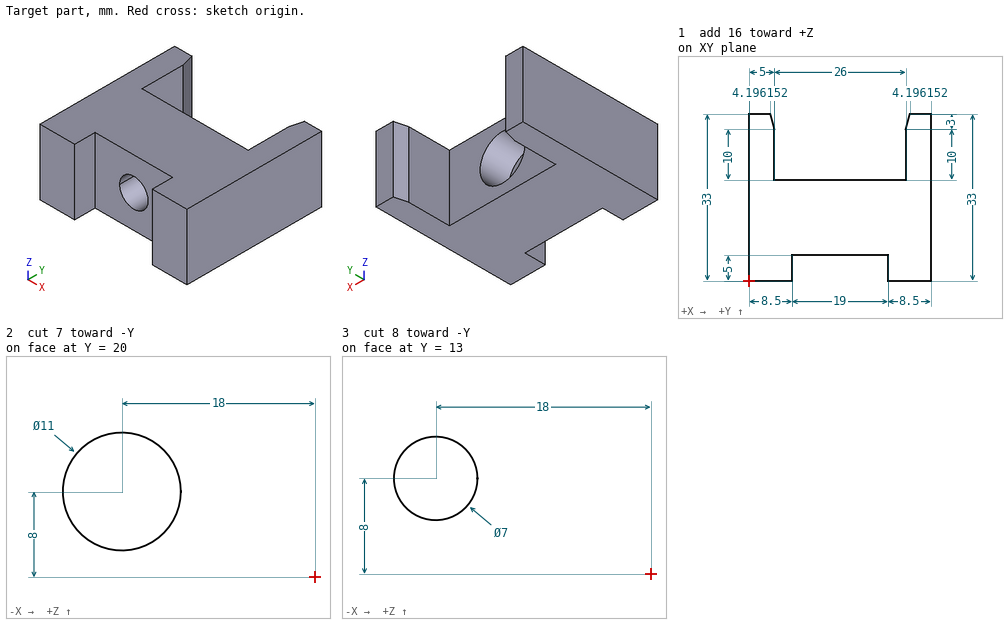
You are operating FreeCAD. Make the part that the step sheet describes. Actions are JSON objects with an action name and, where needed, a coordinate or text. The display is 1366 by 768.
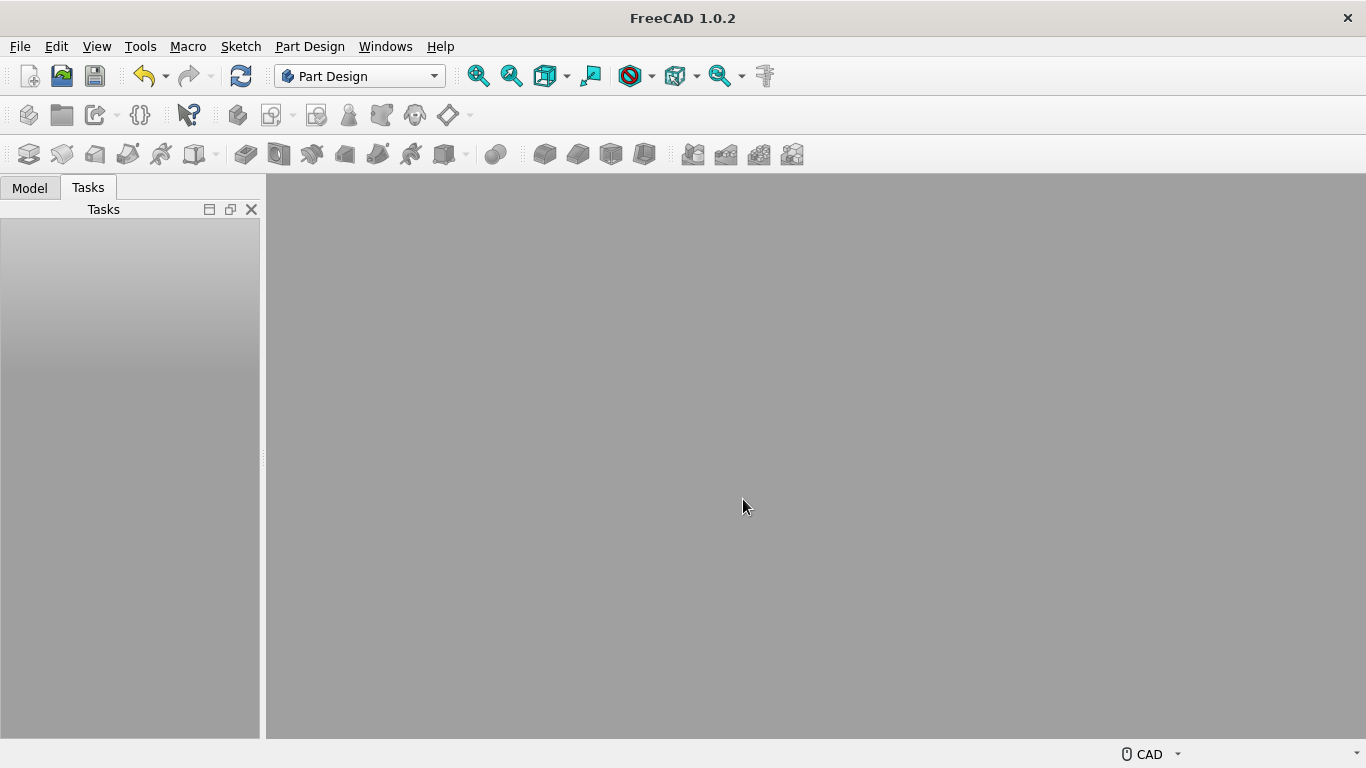
{"action": "left_click", "coordinate": [29, 76]}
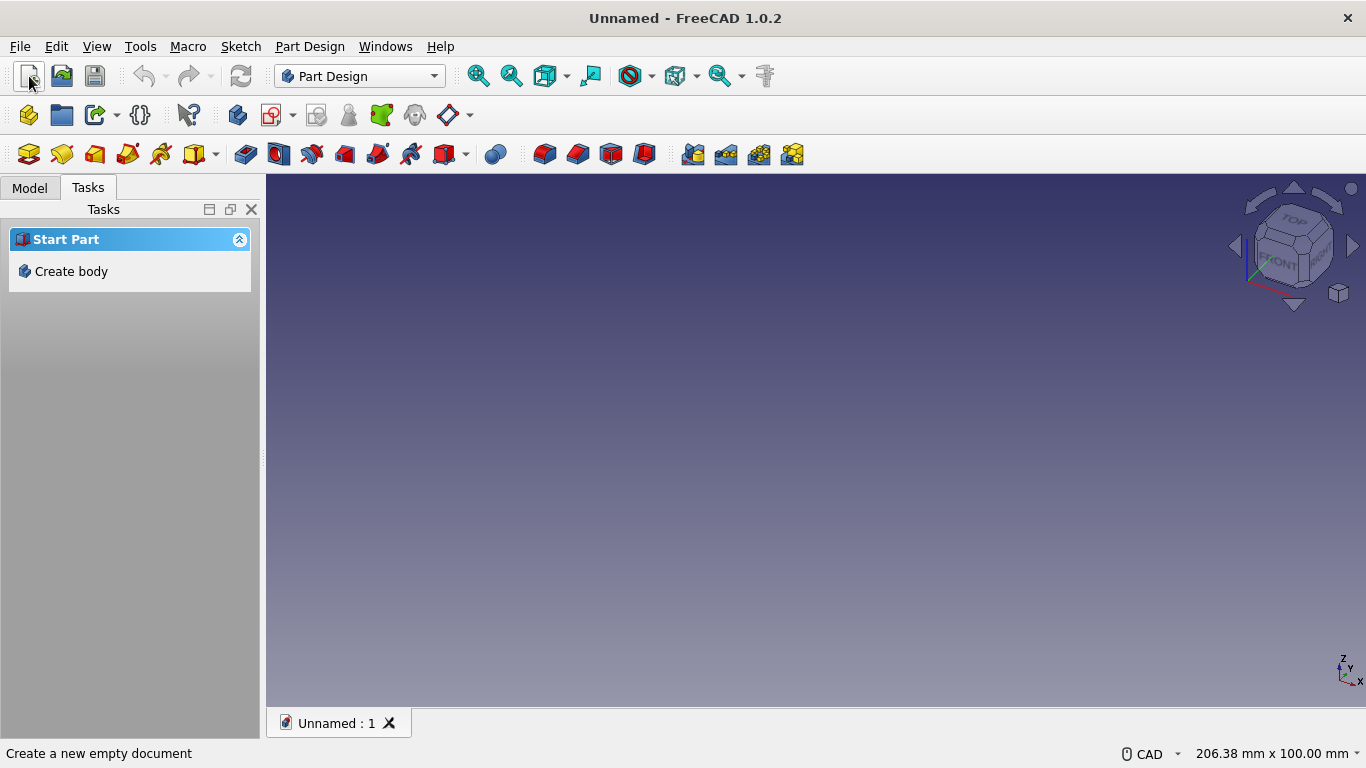
{"action": "left_click", "coordinate": [270, 116]}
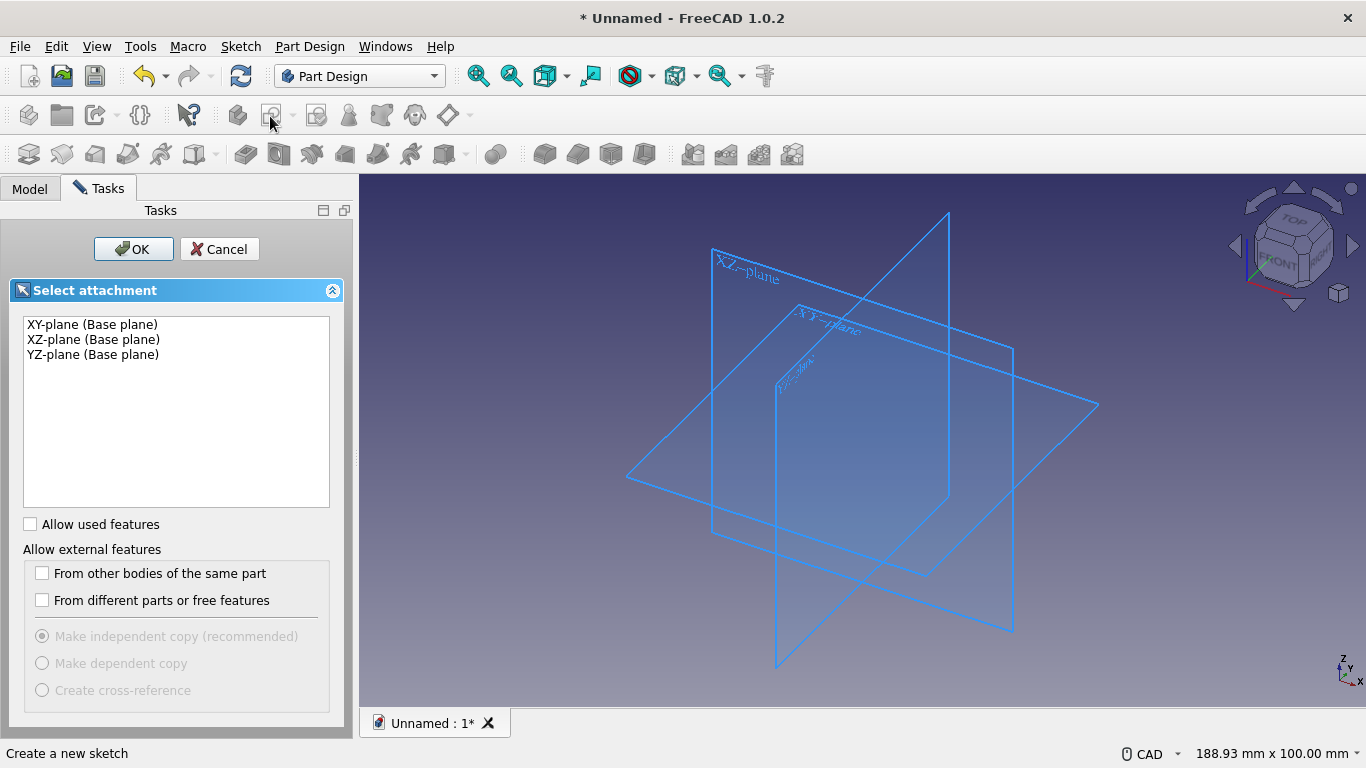
{"action": "left_click", "coordinate": [84, 324]}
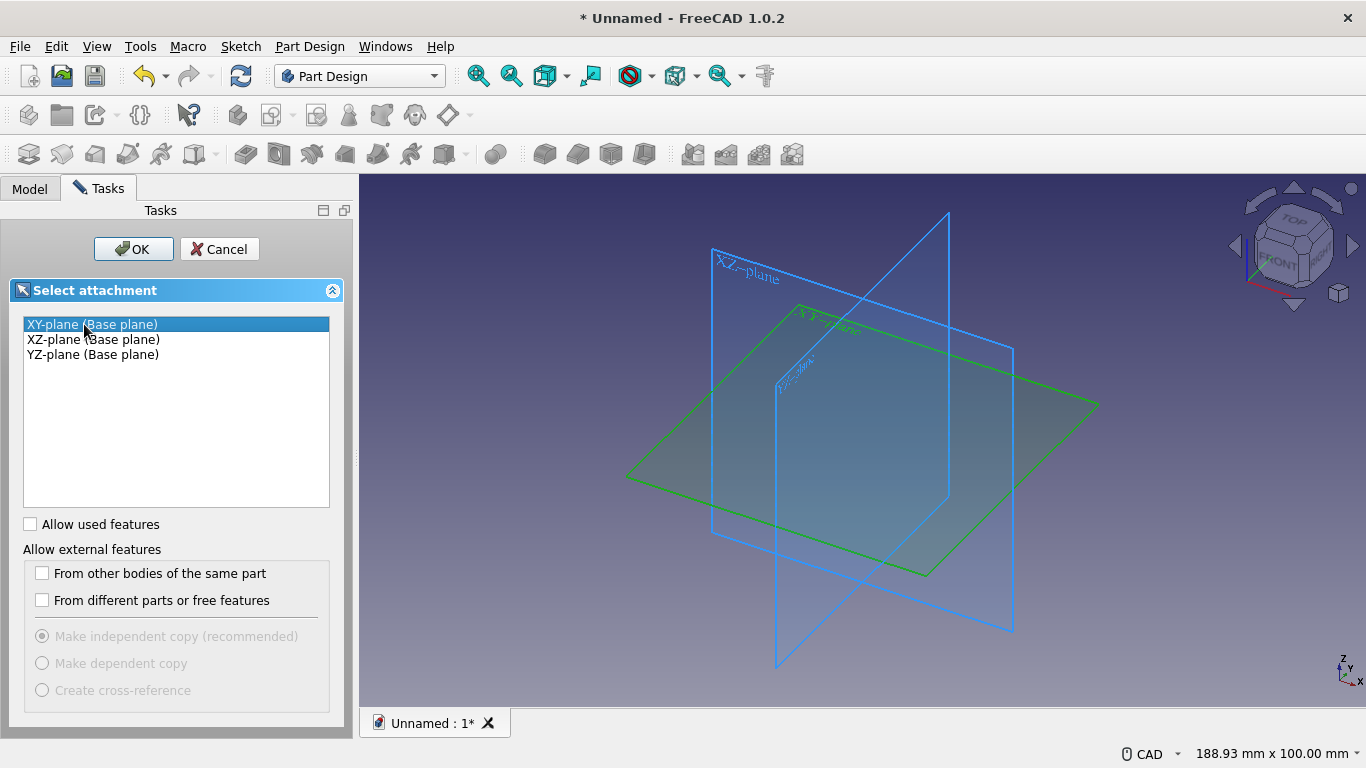
{"action": "left_click", "coordinate": [134, 249]}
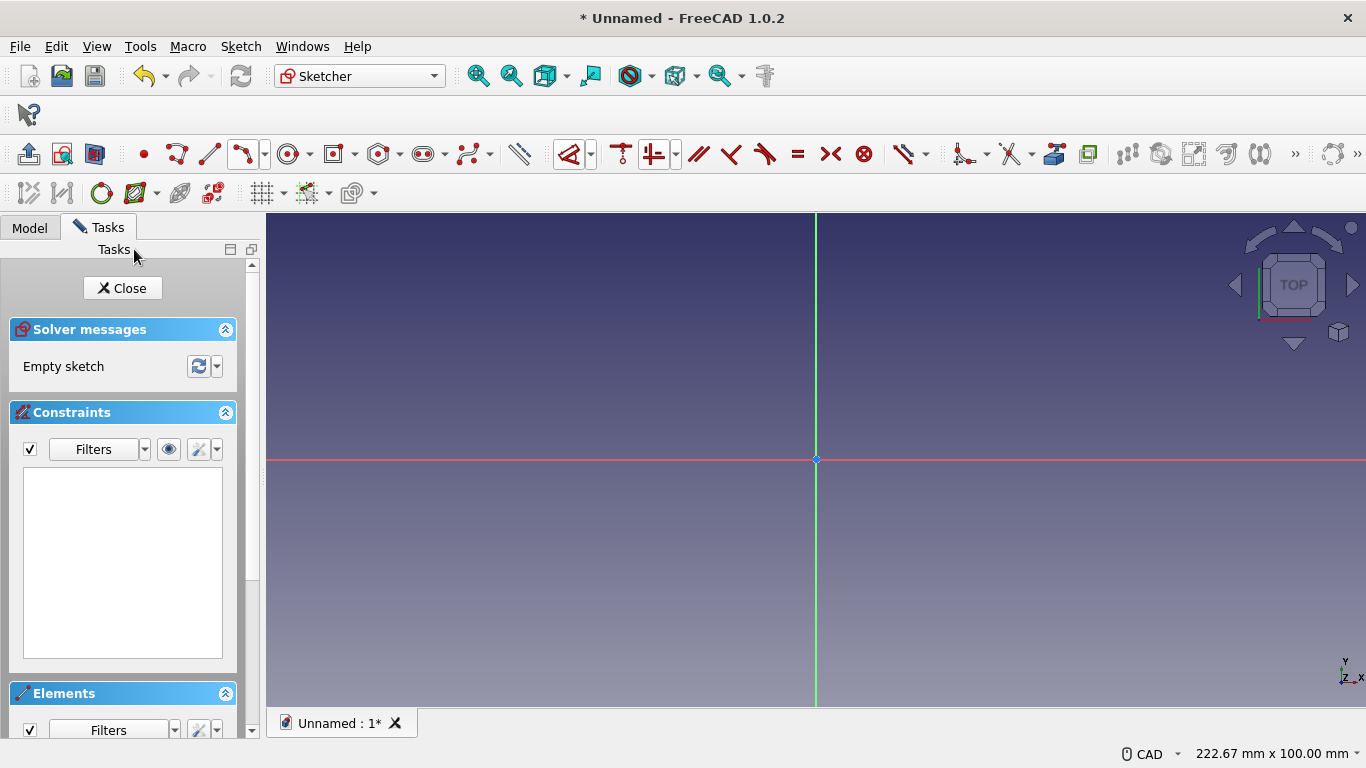
{"action": "scroll", "coordinate": [1096, 279], "scroll_direction": "up", "scroll_amount": 3}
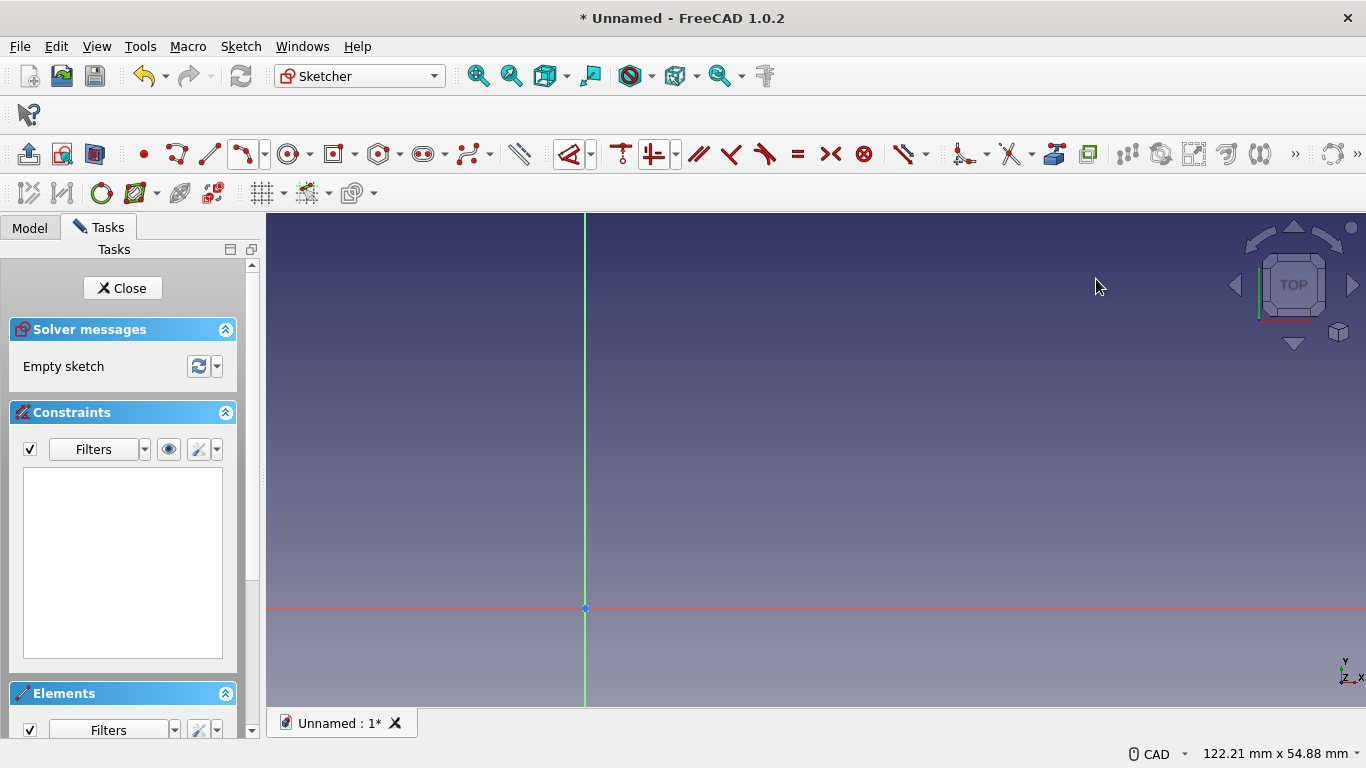
{"action": "left_click", "coordinate": [177, 154]}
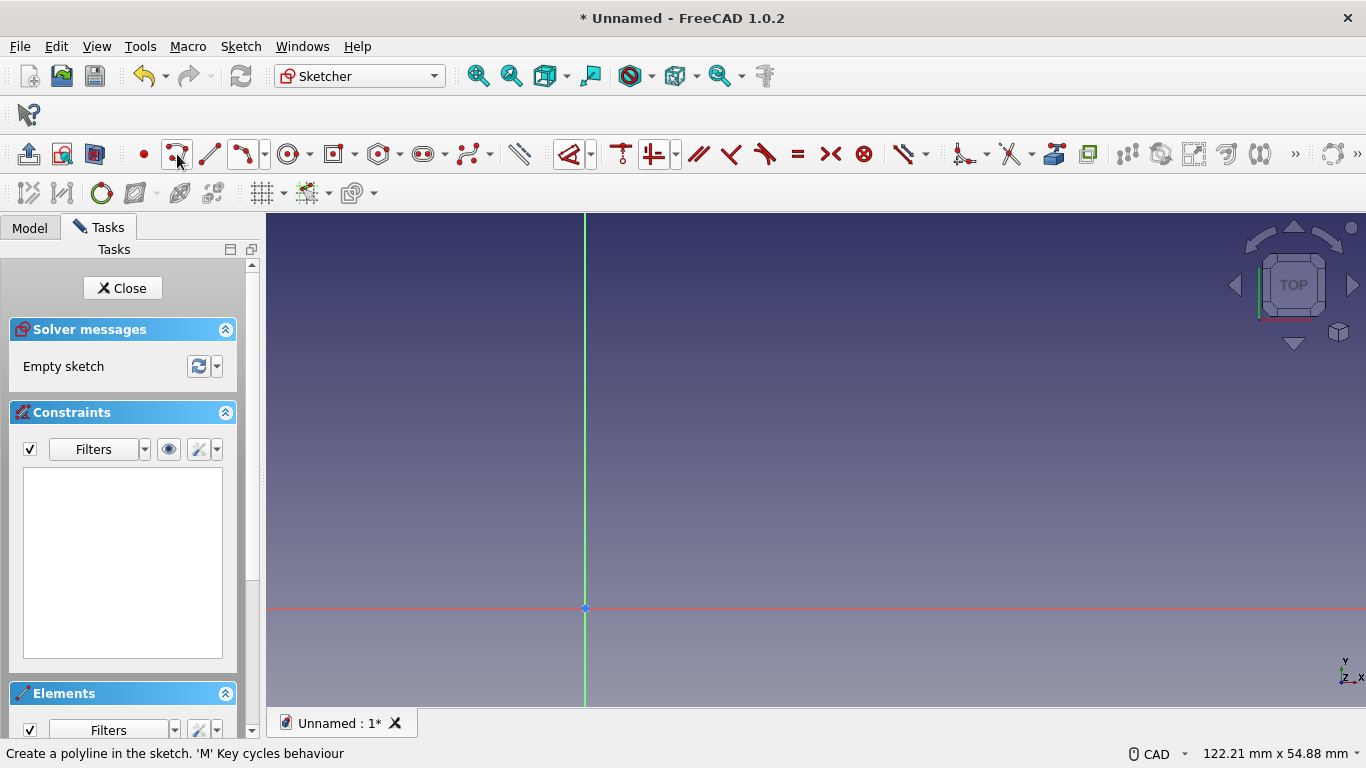
{"action": "left_click", "coordinate": [585, 609]}
{"action": "left_click", "coordinate": [662, 600]}
{"action": "left_click", "coordinate": [662, 564]}
{"action": "left_click", "coordinate": [833, 564]}
{"action": "left_click", "coordinate": [833, 609]}
{"action": "left_click", "coordinate": [909, 600]}
{"action": "left_click", "coordinate": [909, 312]}
{"action": "left_click", "coordinate": [871, 312]}
{"action": "left_click", "coordinate": [864, 339]}
{"action": "left_click", "coordinate": [864, 429]}
{"action": "left_click", "coordinate": [630, 429]}
{"action": "left_click", "coordinate": [630, 339]}
{"action": "left_click", "coordinate": [623, 312]}
{"action": "left_click", "coordinate": [594, 312]}
{"action": "left_click", "coordinate": [585, 609]}
{"action": "key", "text": "Escape"}
{"action": "key", "text": "Escape"}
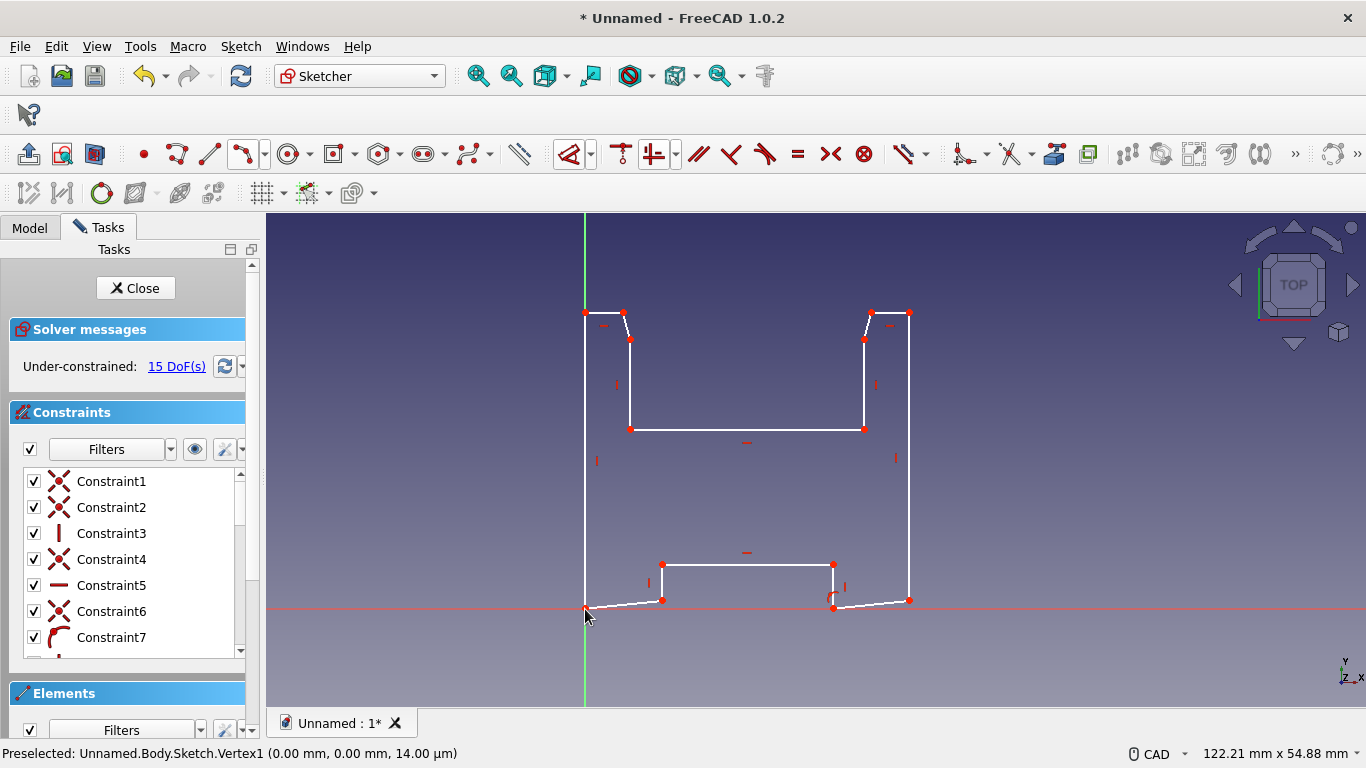
{"action": "left_click", "coordinate": [608, 606]}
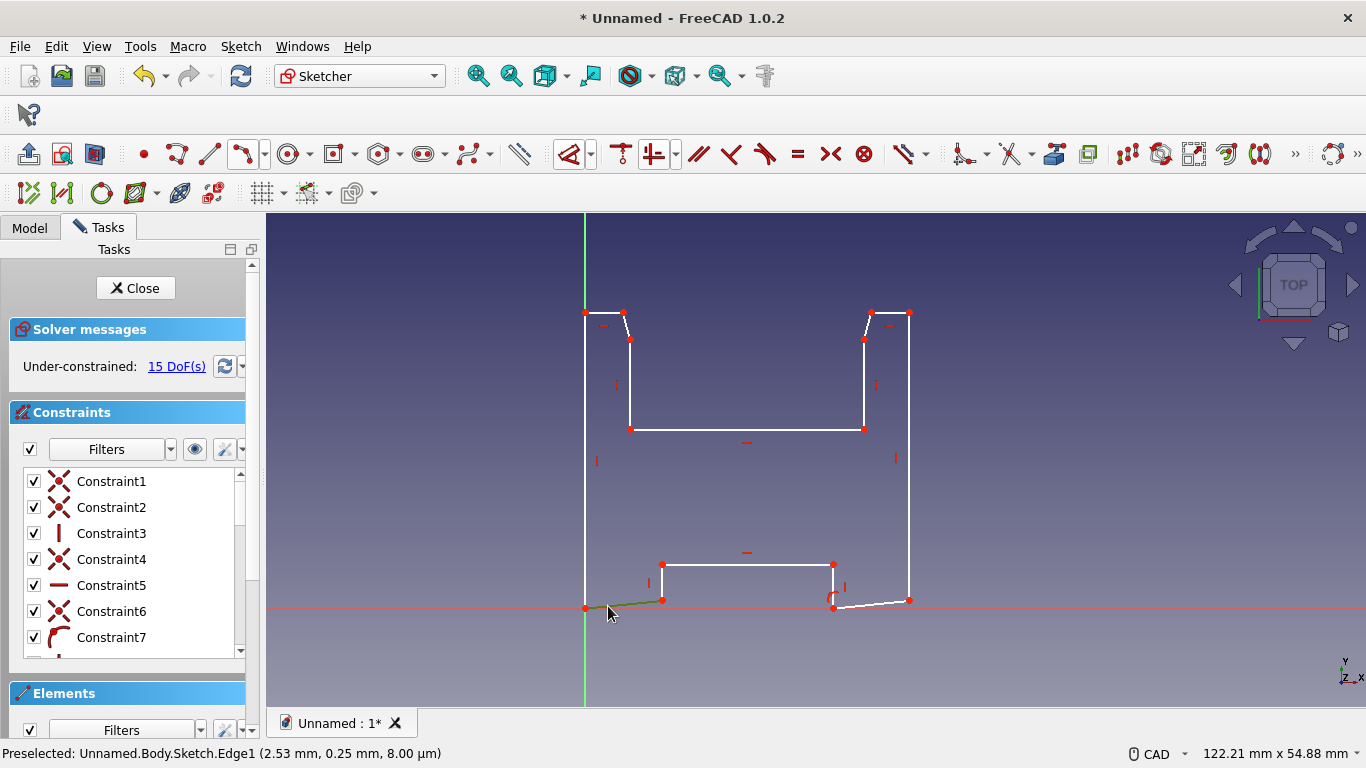
{"action": "left_click", "coordinate": [676, 154]}